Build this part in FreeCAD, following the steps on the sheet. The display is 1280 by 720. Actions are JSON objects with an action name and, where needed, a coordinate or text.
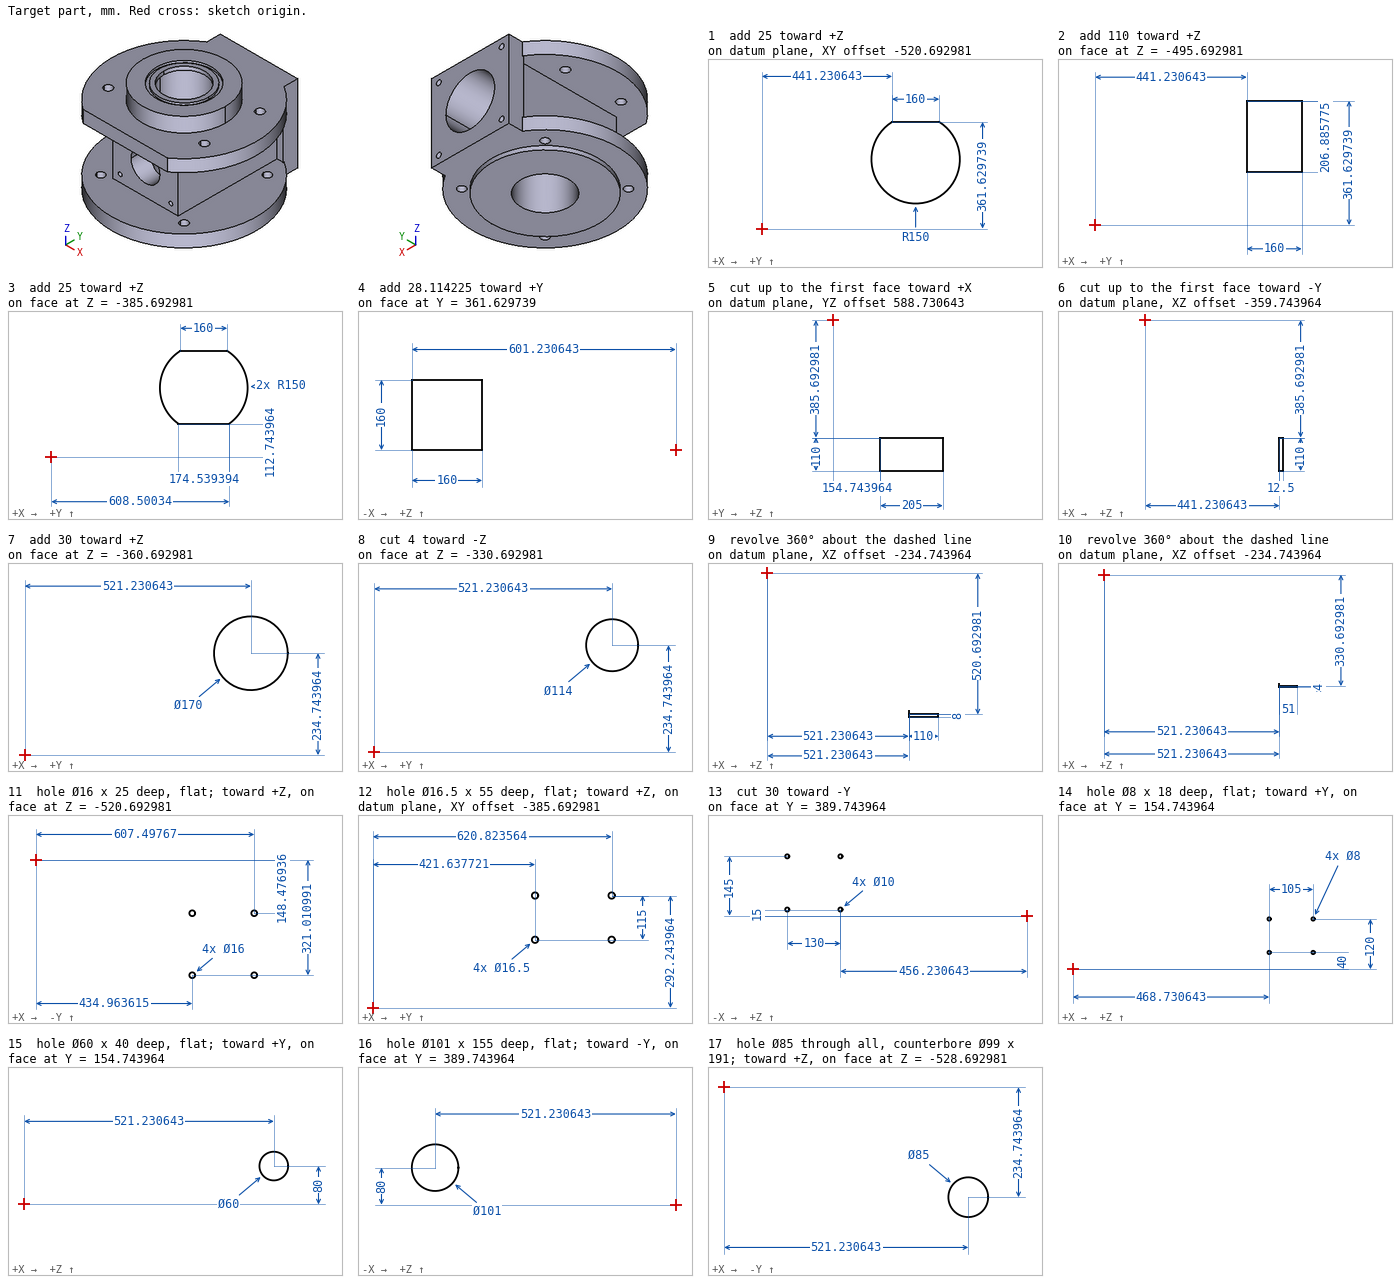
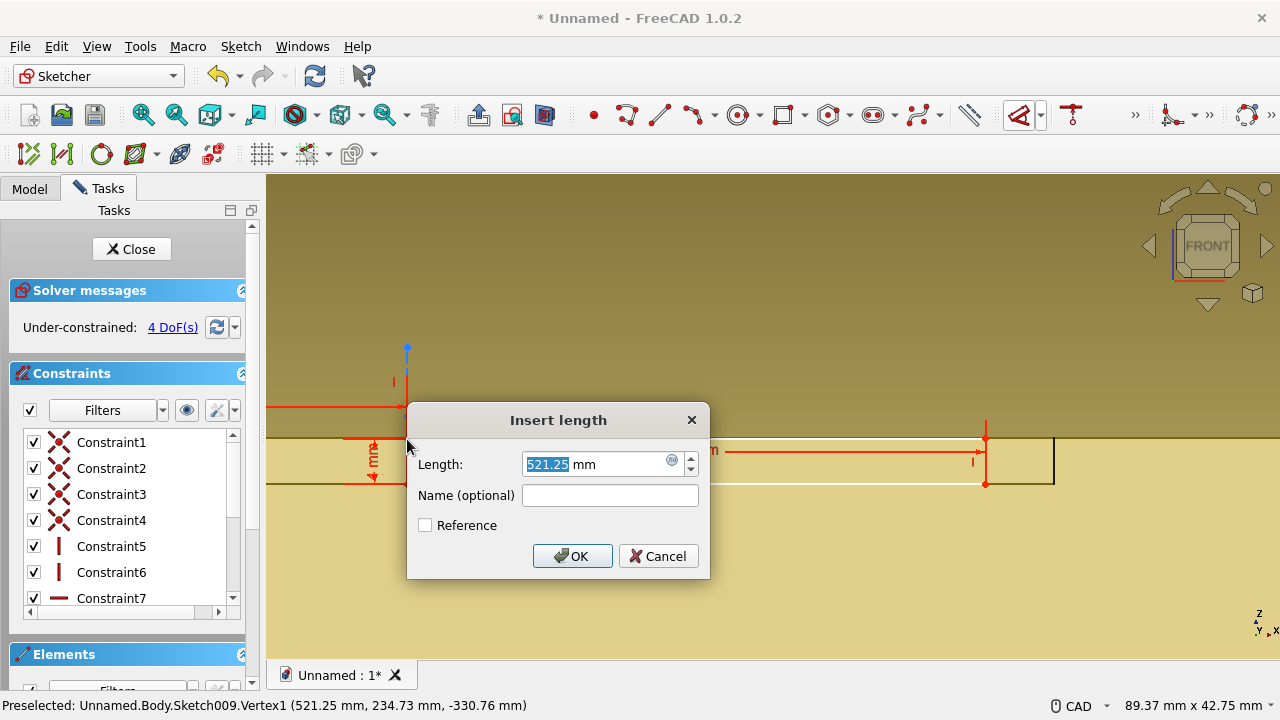
{"action": "type", "text": "521.230643"}
{"action": "key", "text": "Return"}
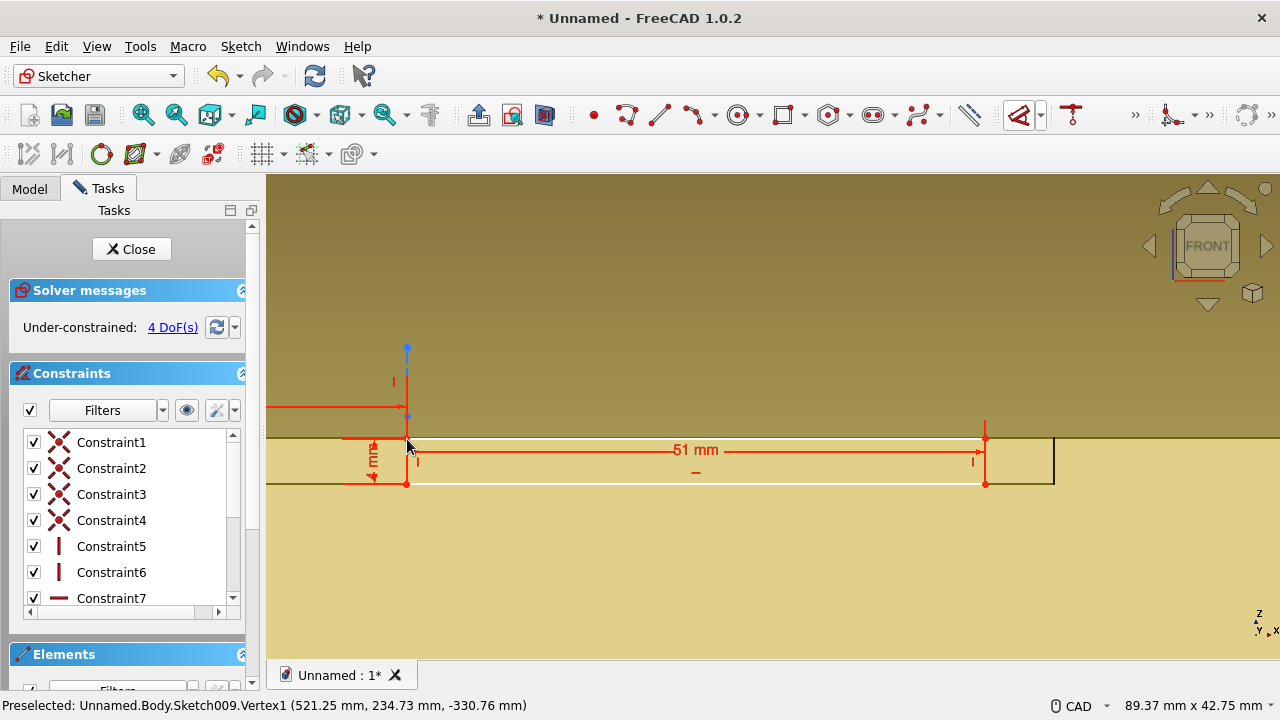
{"action": "left_click", "coordinate": [407, 439]}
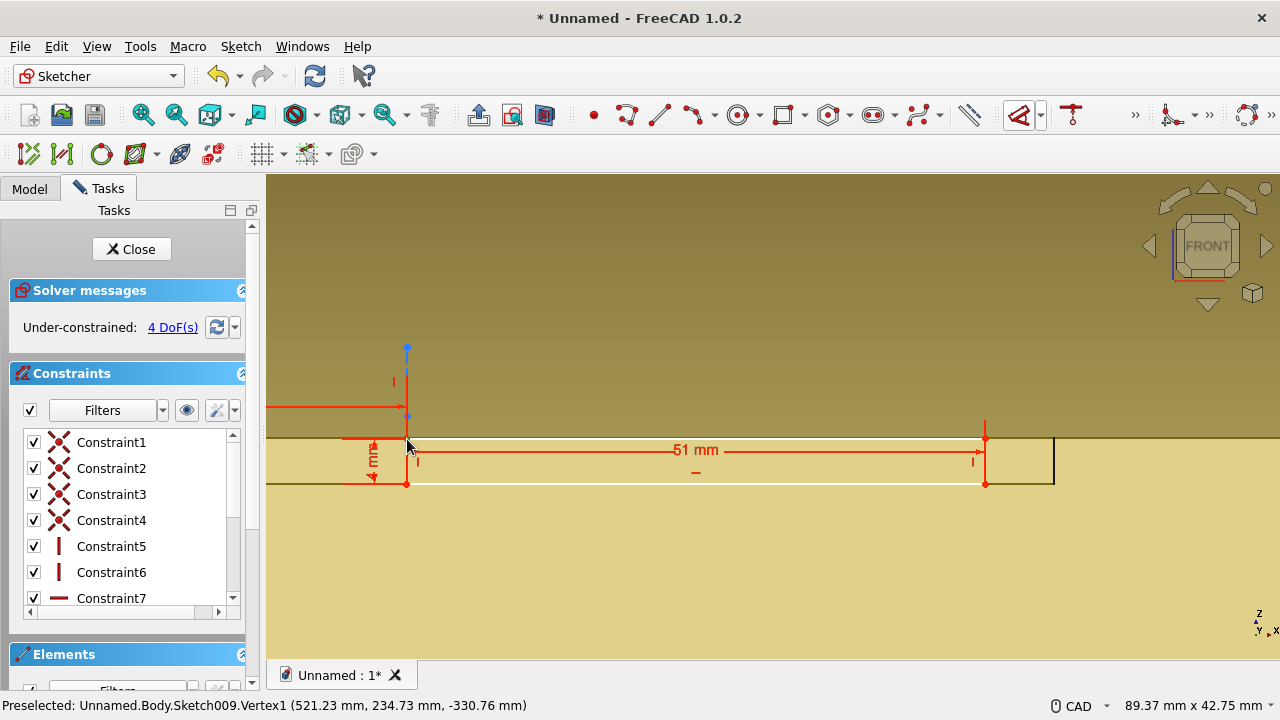
{"action": "left_click", "coordinate": [1040, 116]}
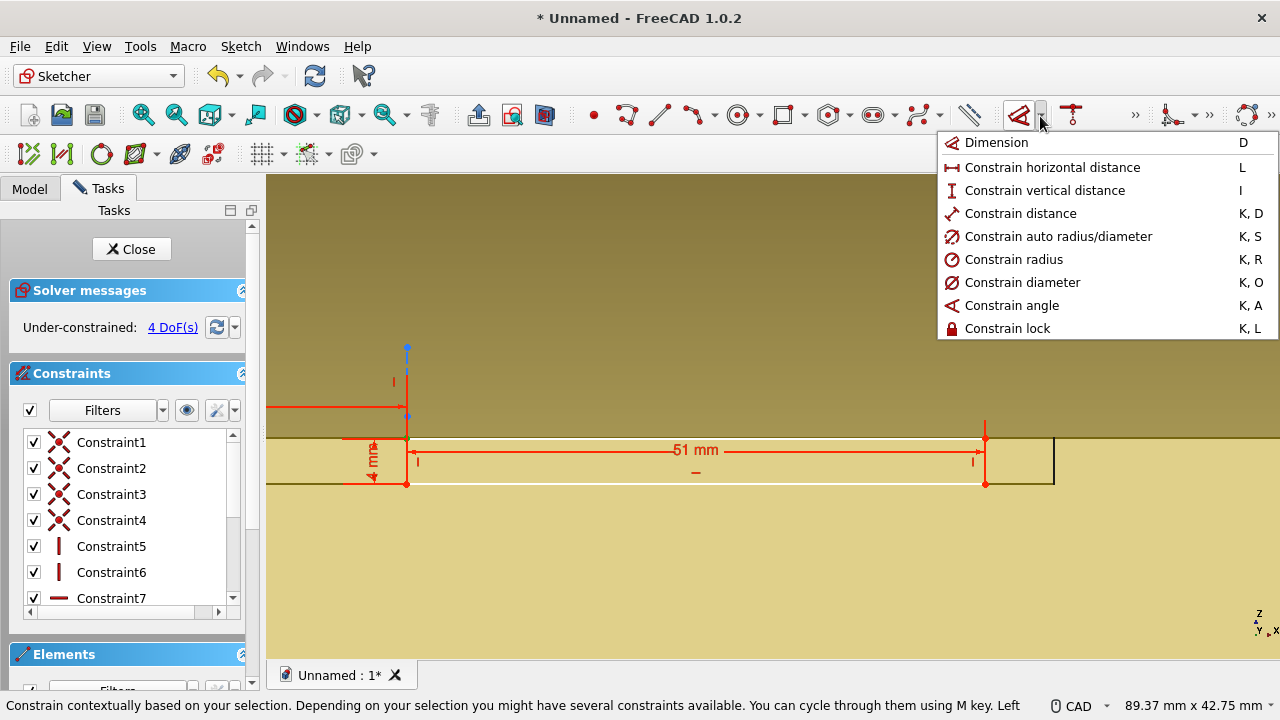
{"action": "left_click", "coordinate": [1108, 190]}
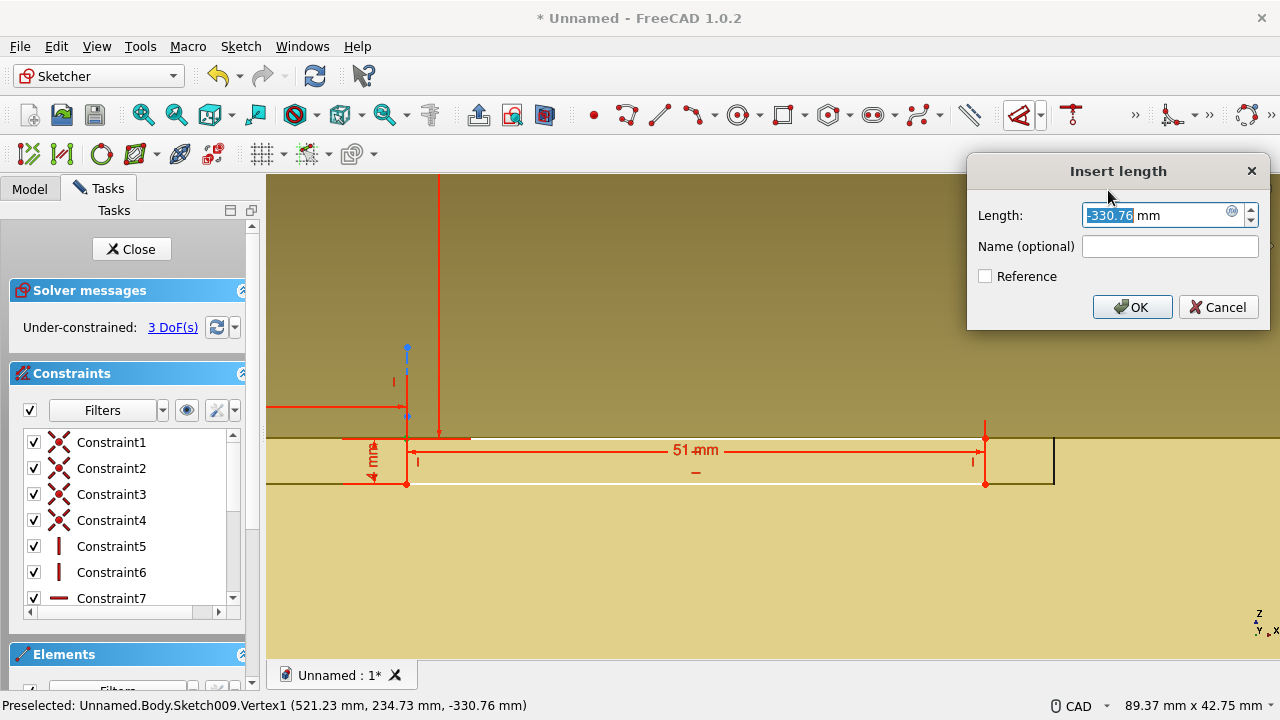
{"action": "type", "text": "-330.692981"}
{"action": "key", "text": "Return"}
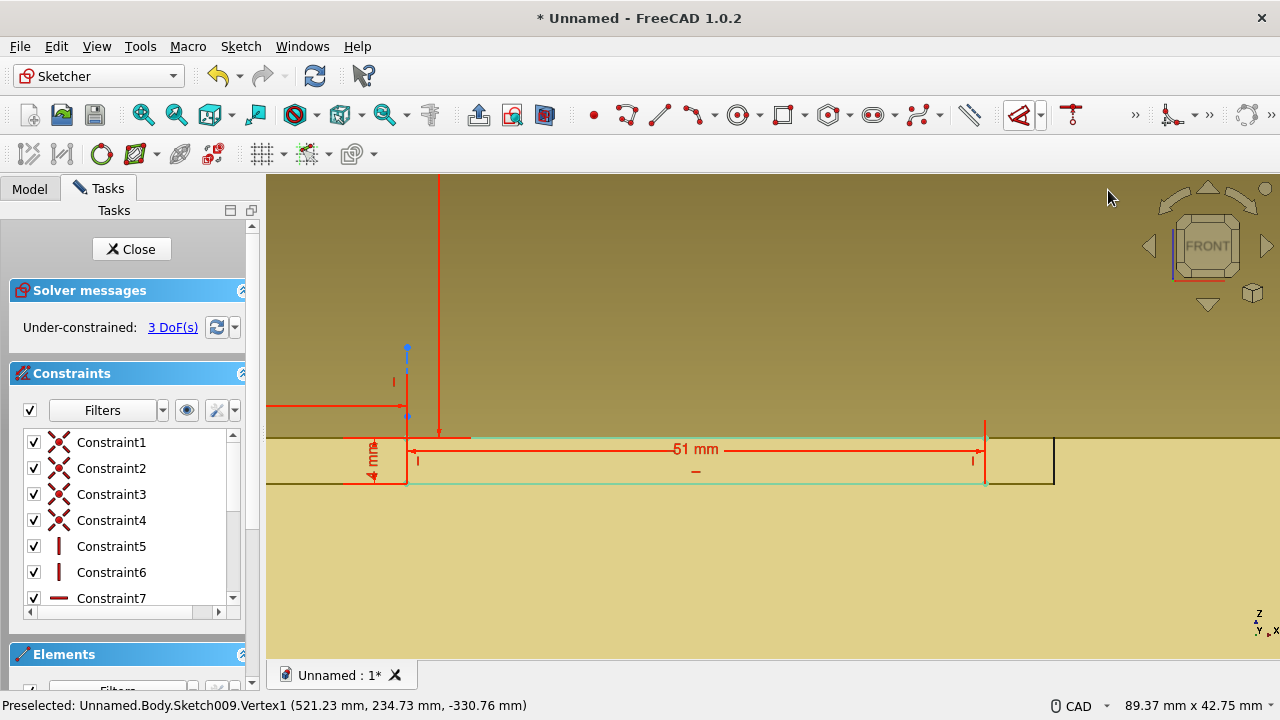
{"action": "left_click", "coordinate": [407, 416]}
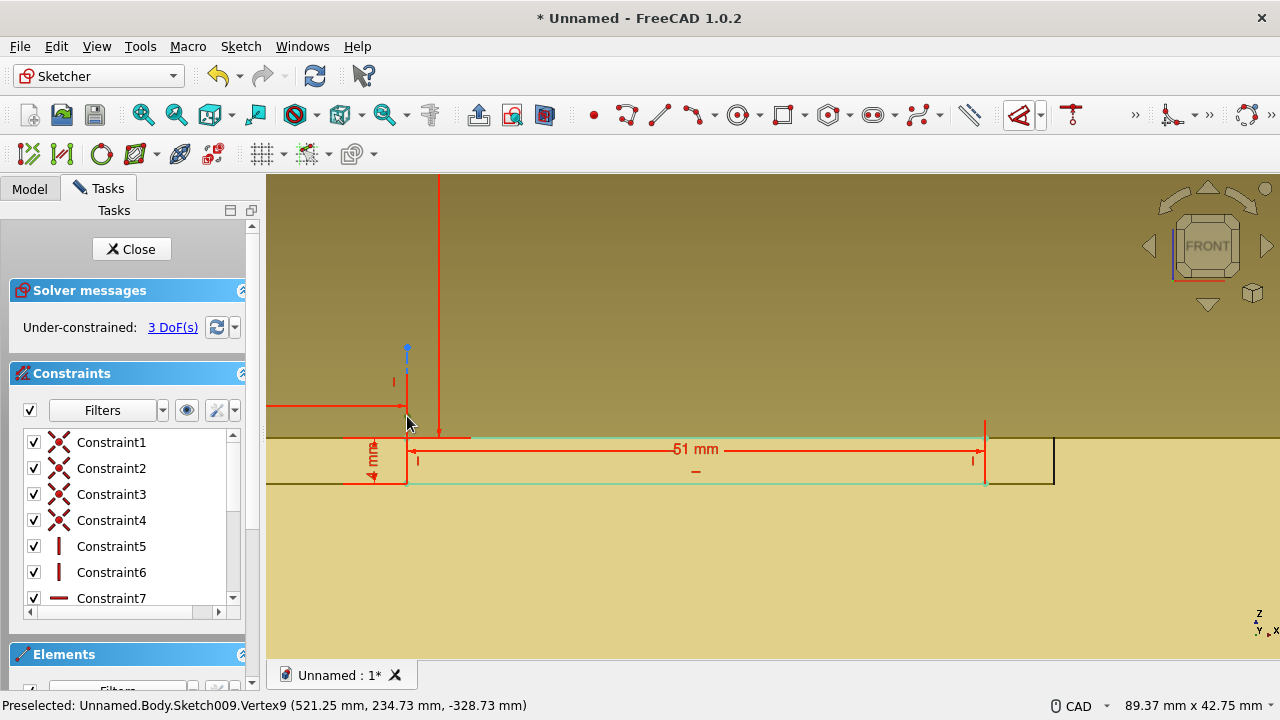
{"action": "left_click", "coordinate": [1040, 116]}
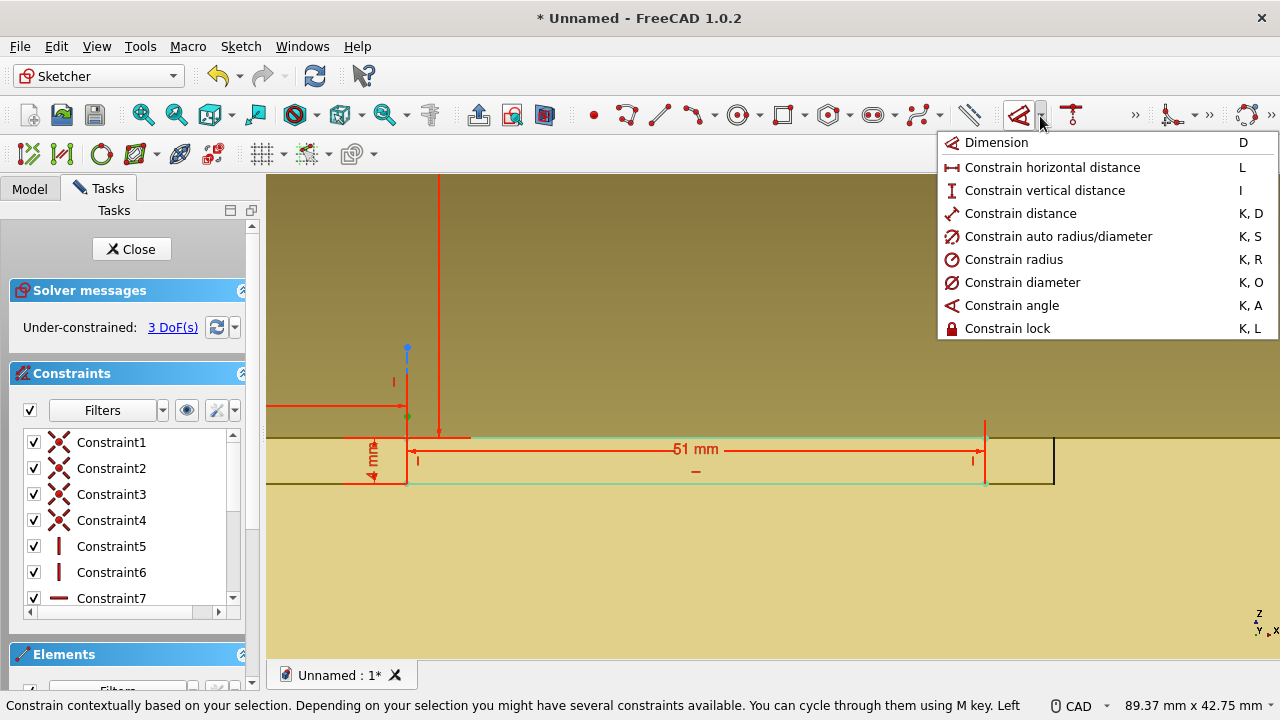
{"action": "left_click", "coordinate": [1108, 168]}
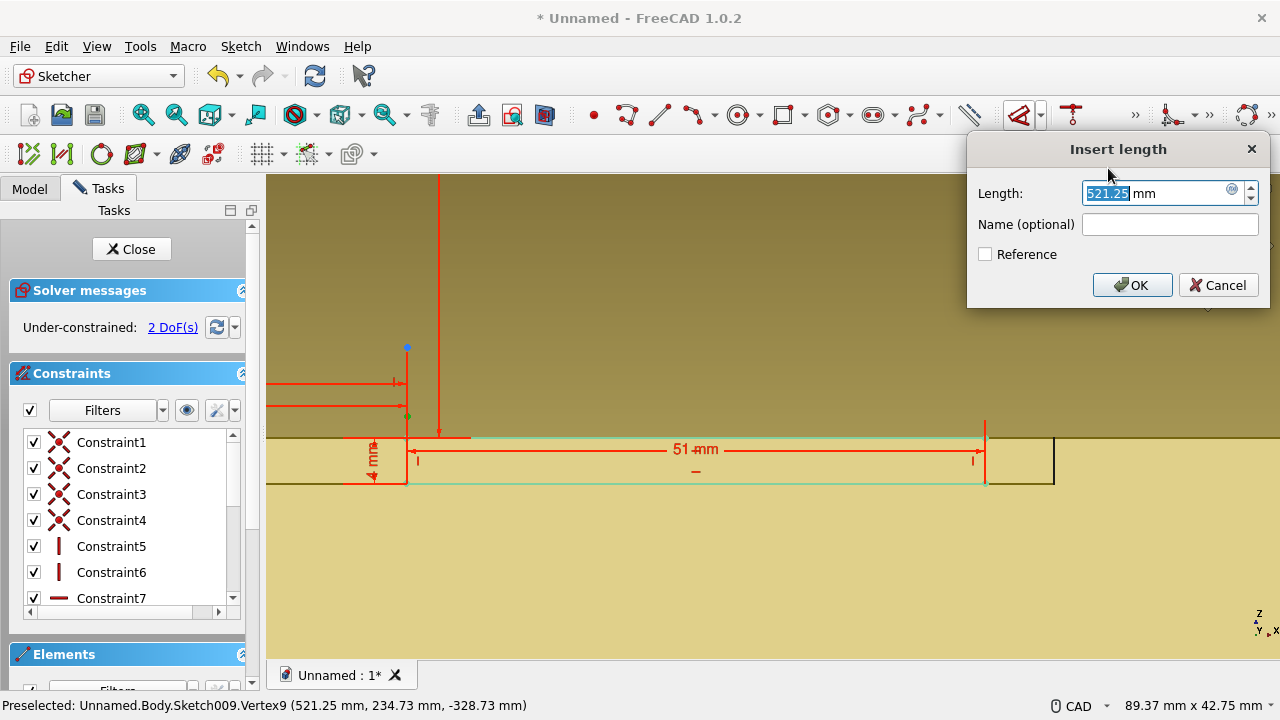
{"action": "type", "text": "521.230643"}
{"action": "key", "text": "Return"}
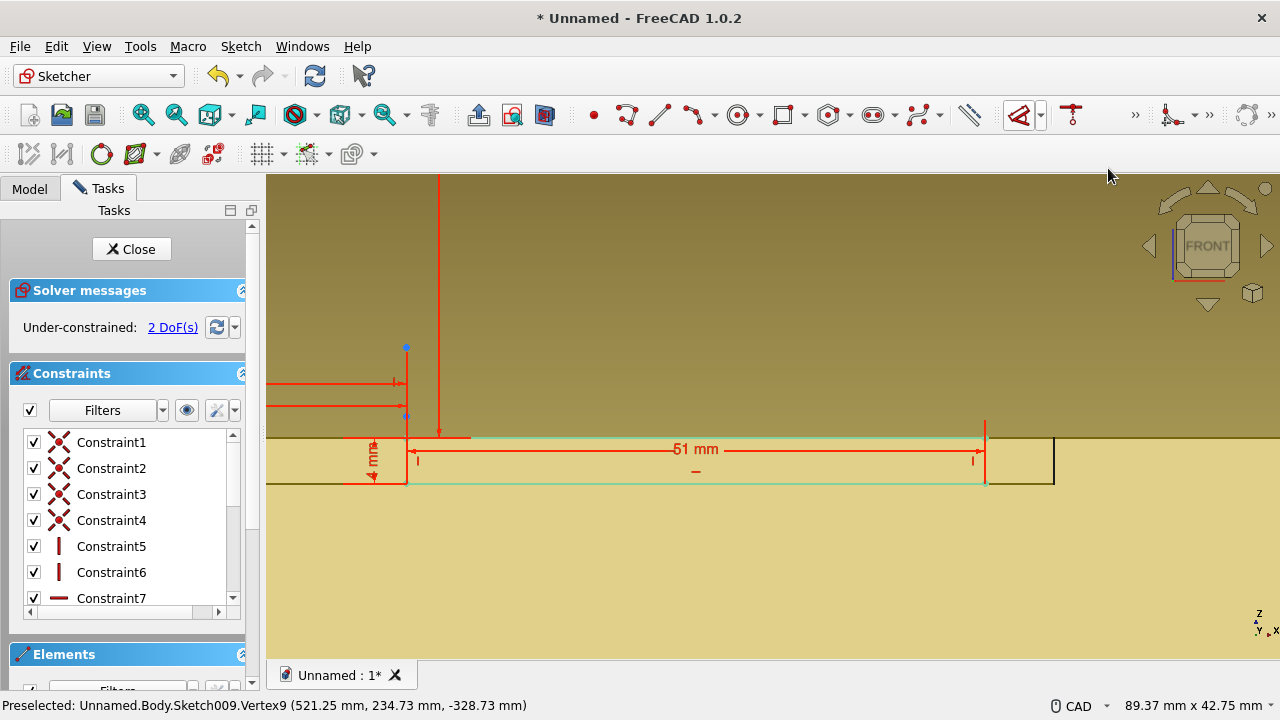
{"action": "left_click", "coordinate": [132, 249]}